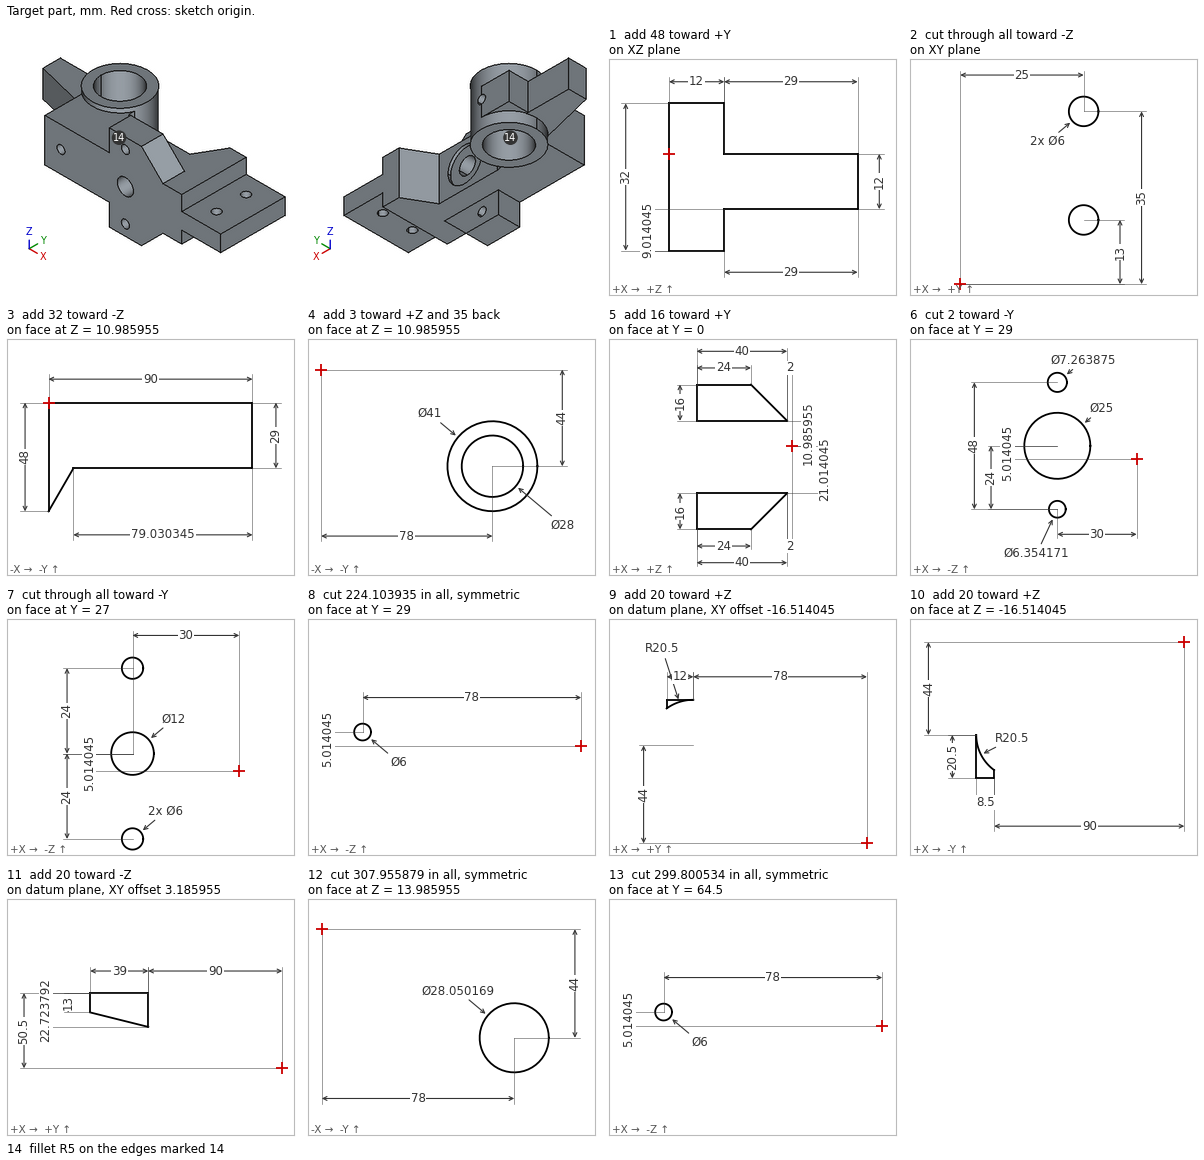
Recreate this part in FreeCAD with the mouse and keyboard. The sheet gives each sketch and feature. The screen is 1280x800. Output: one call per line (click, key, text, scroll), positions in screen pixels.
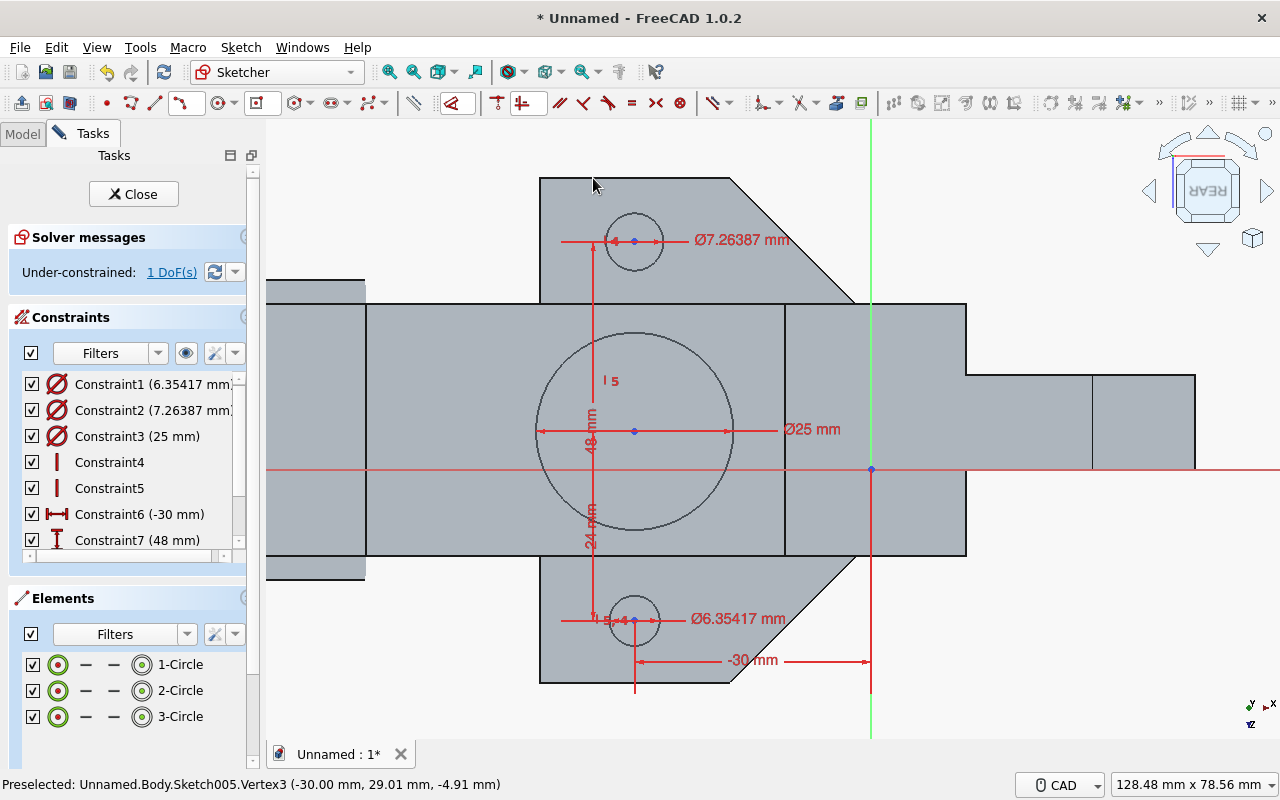
click(635, 431)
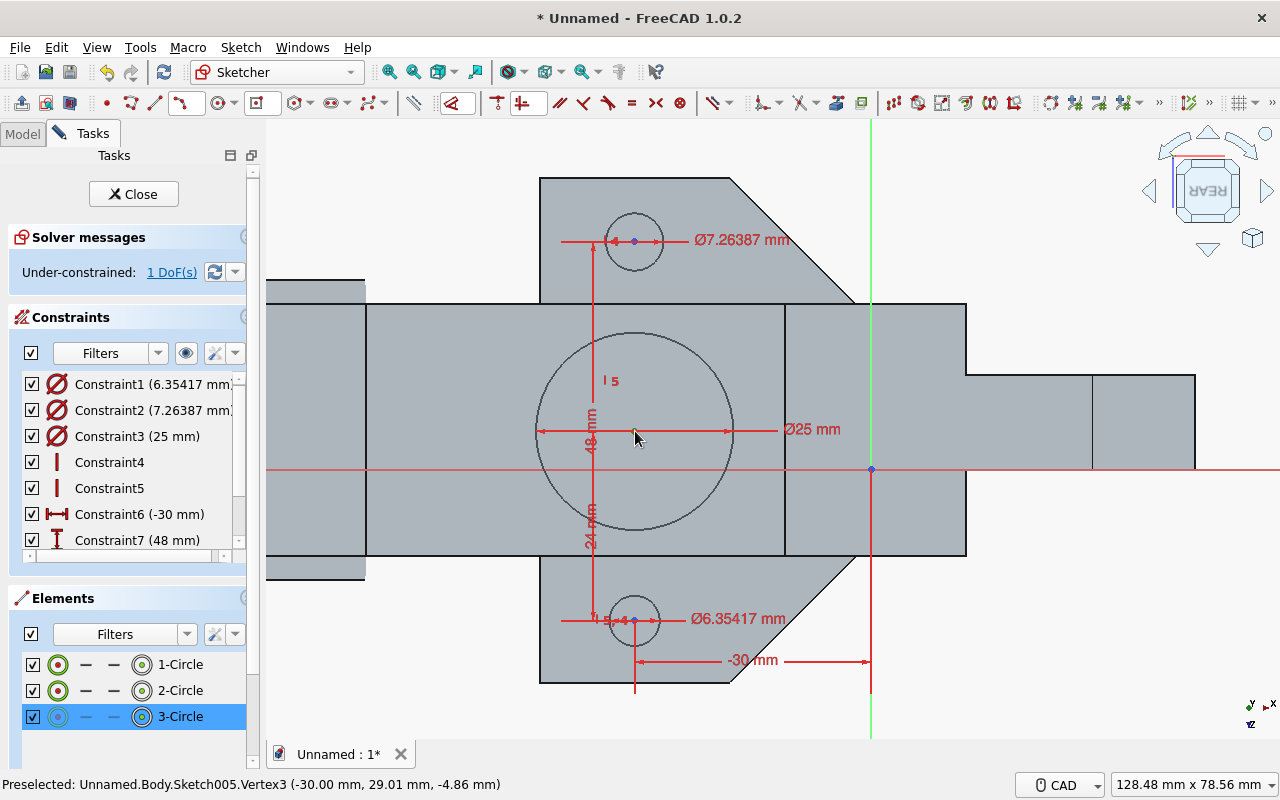
key(i)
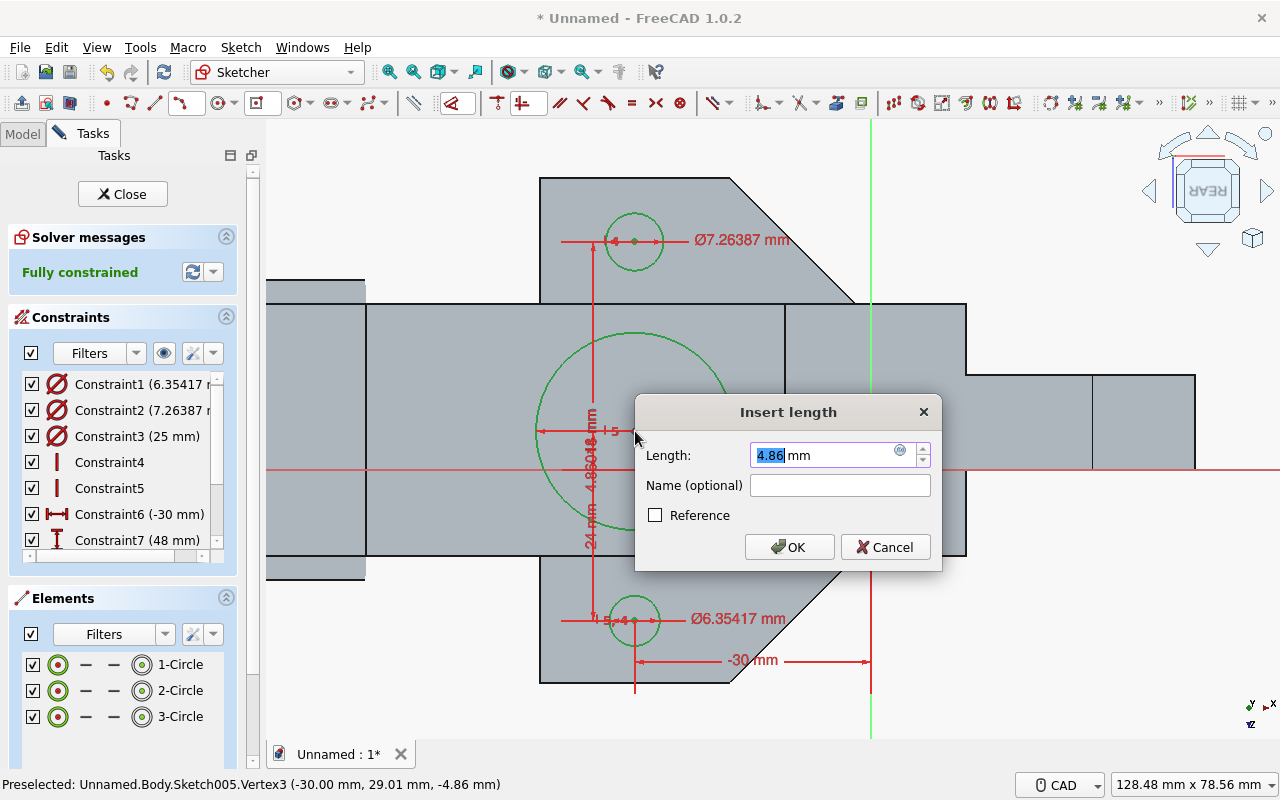
text(5.014045)
key(Return)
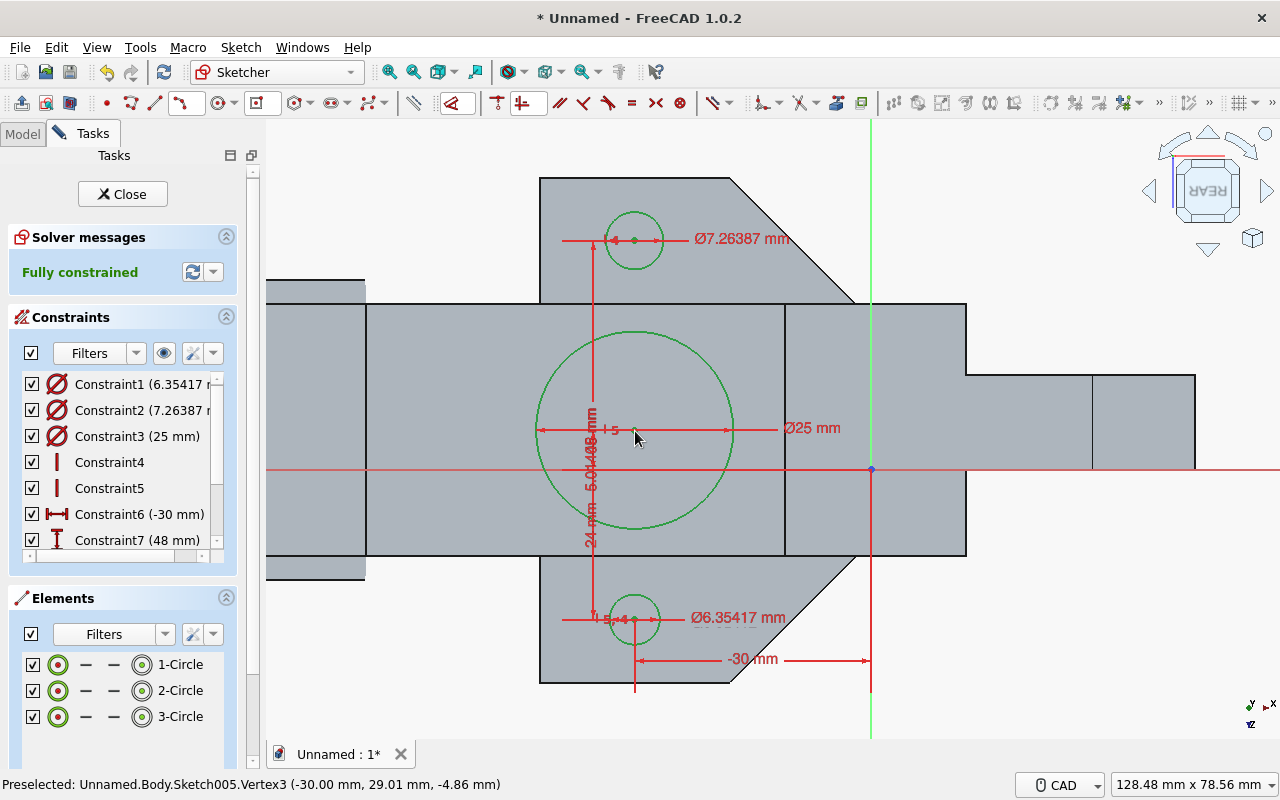
click(123, 194)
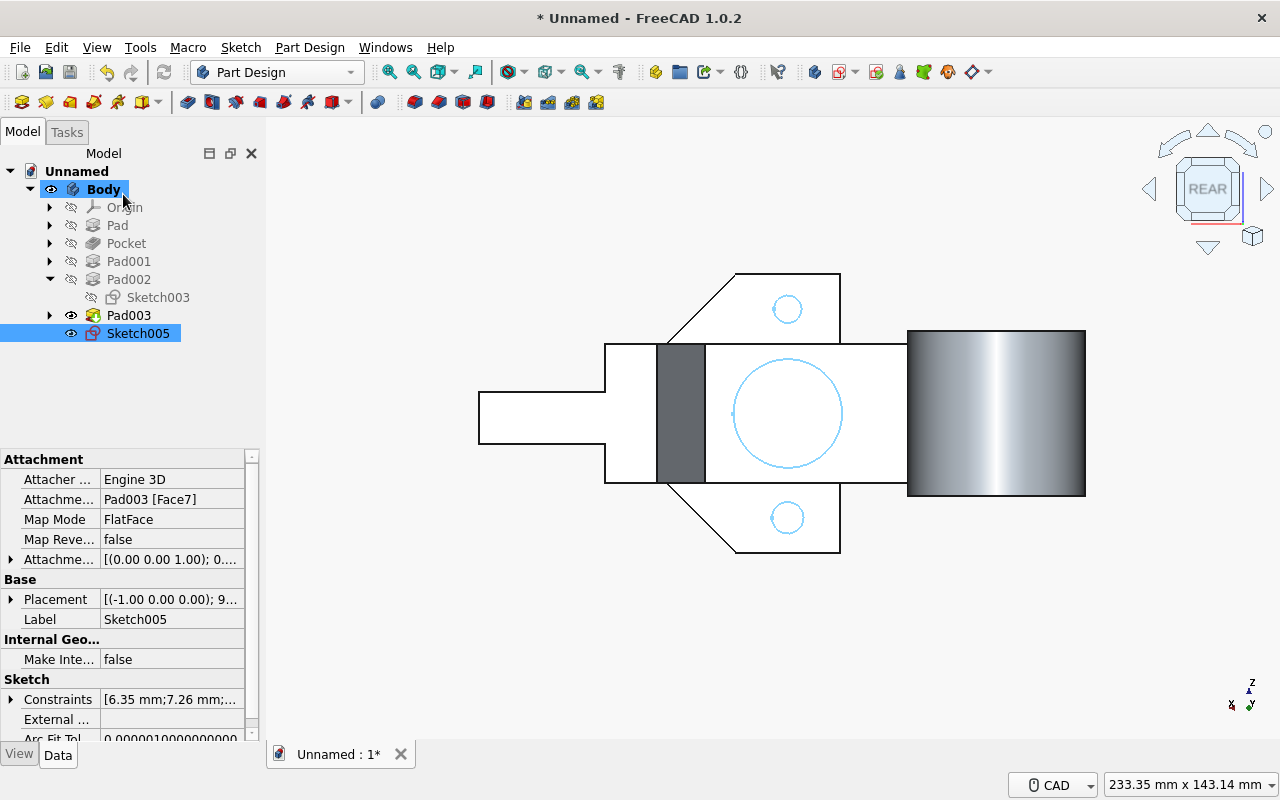
click(188, 102)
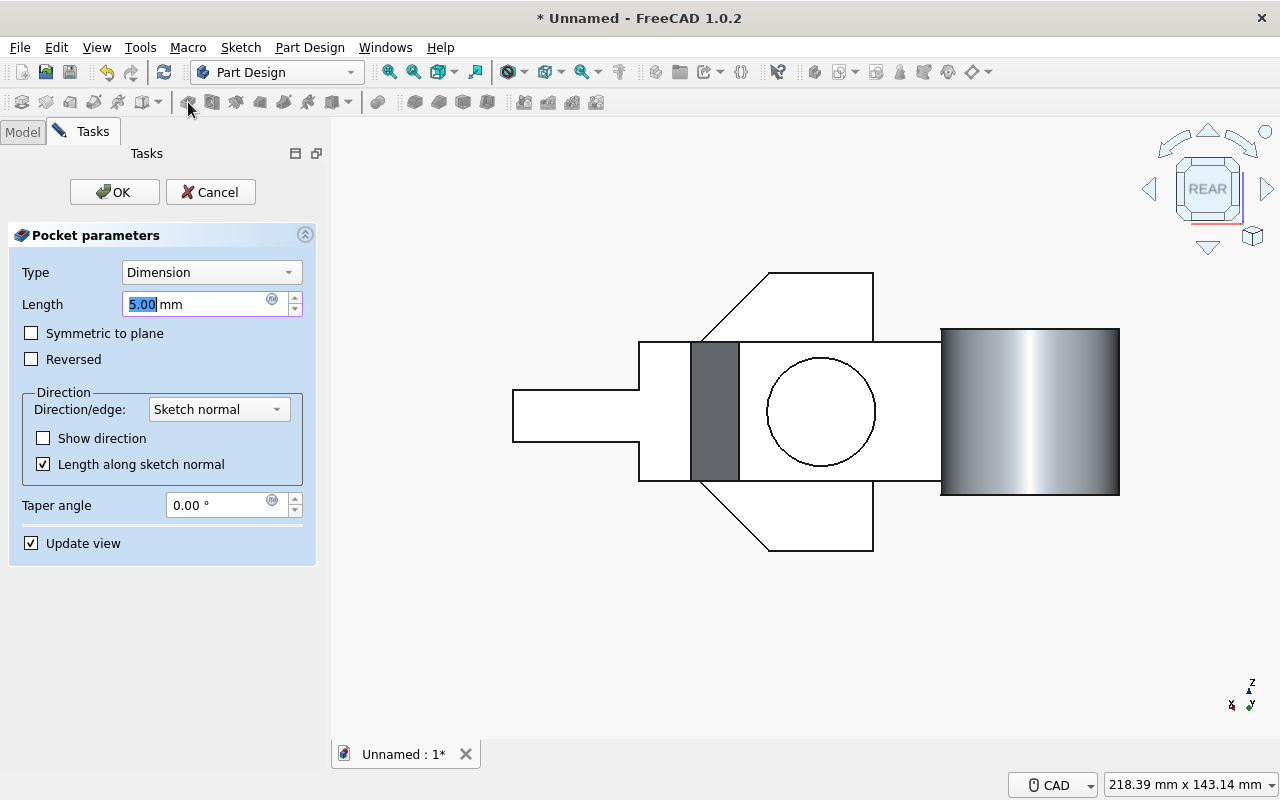
text(2)
key(Tab)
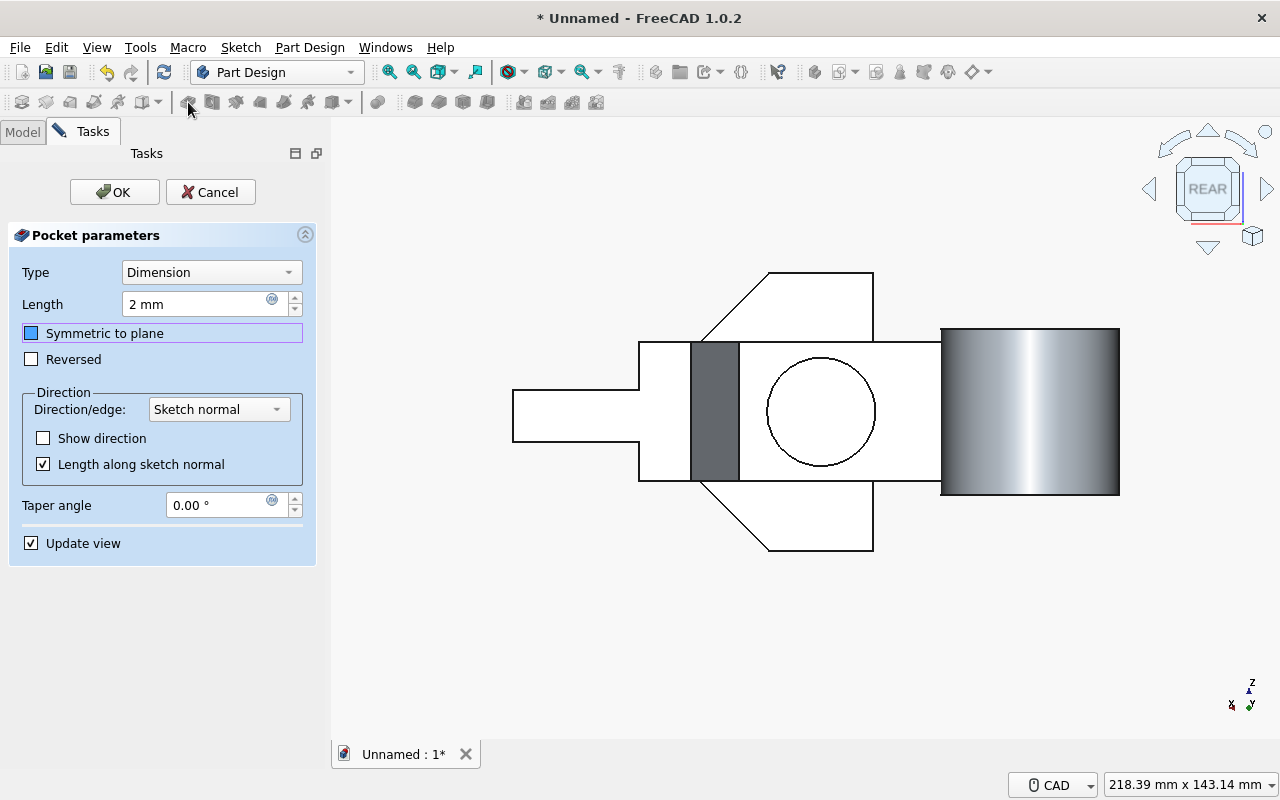
click(115, 192)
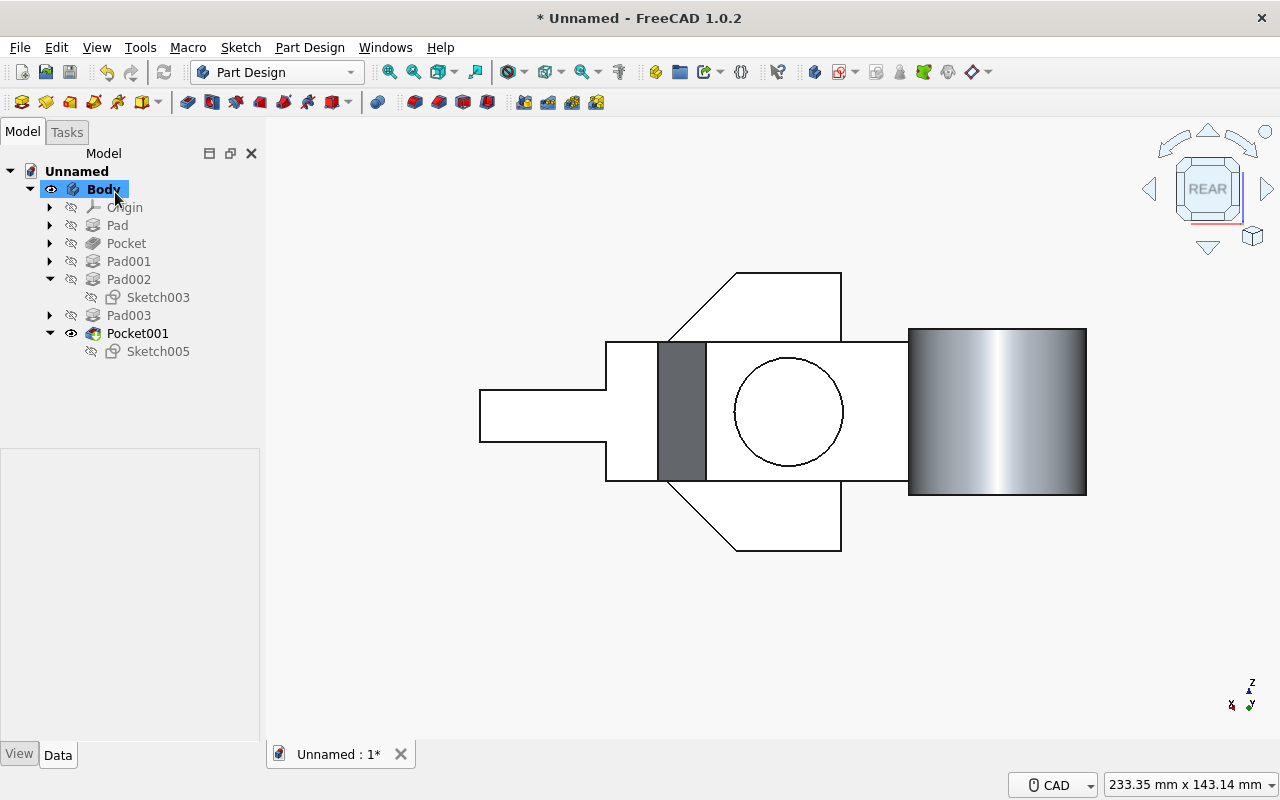
click(789, 411)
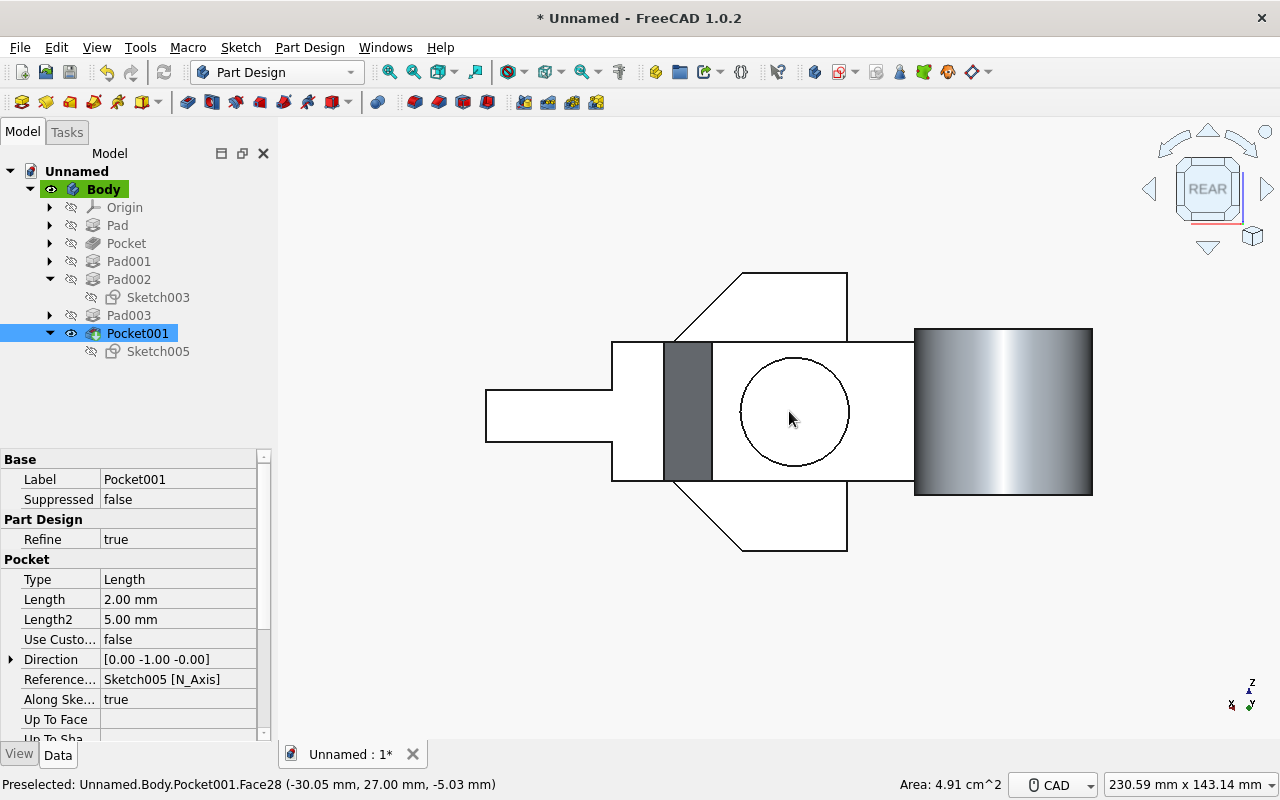
click(840, 72)